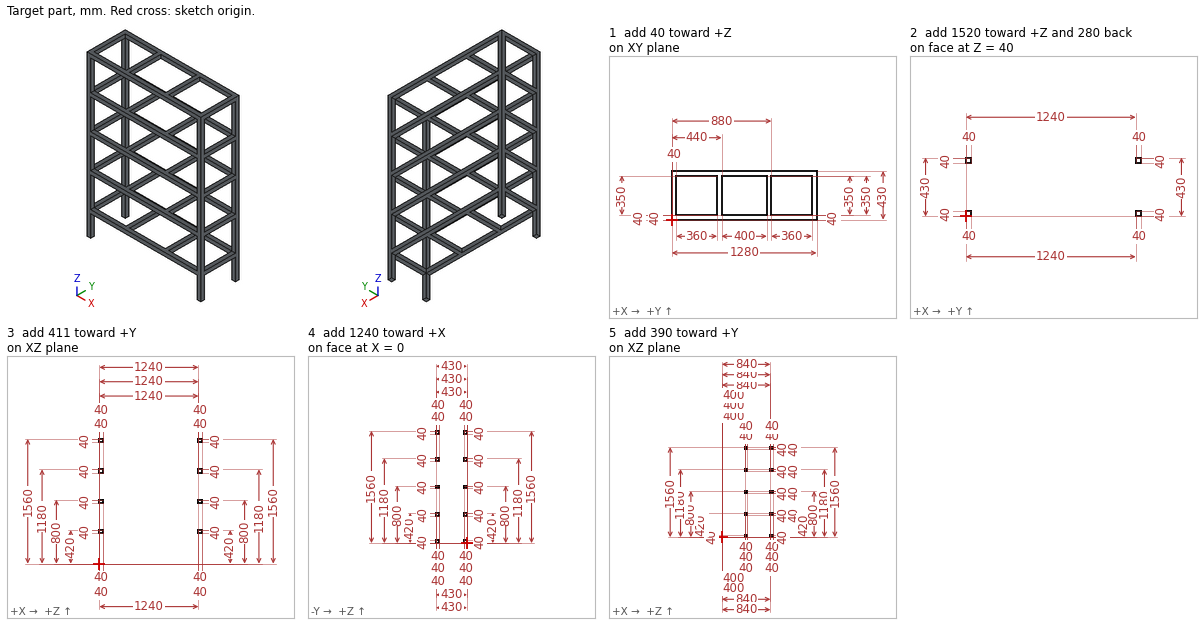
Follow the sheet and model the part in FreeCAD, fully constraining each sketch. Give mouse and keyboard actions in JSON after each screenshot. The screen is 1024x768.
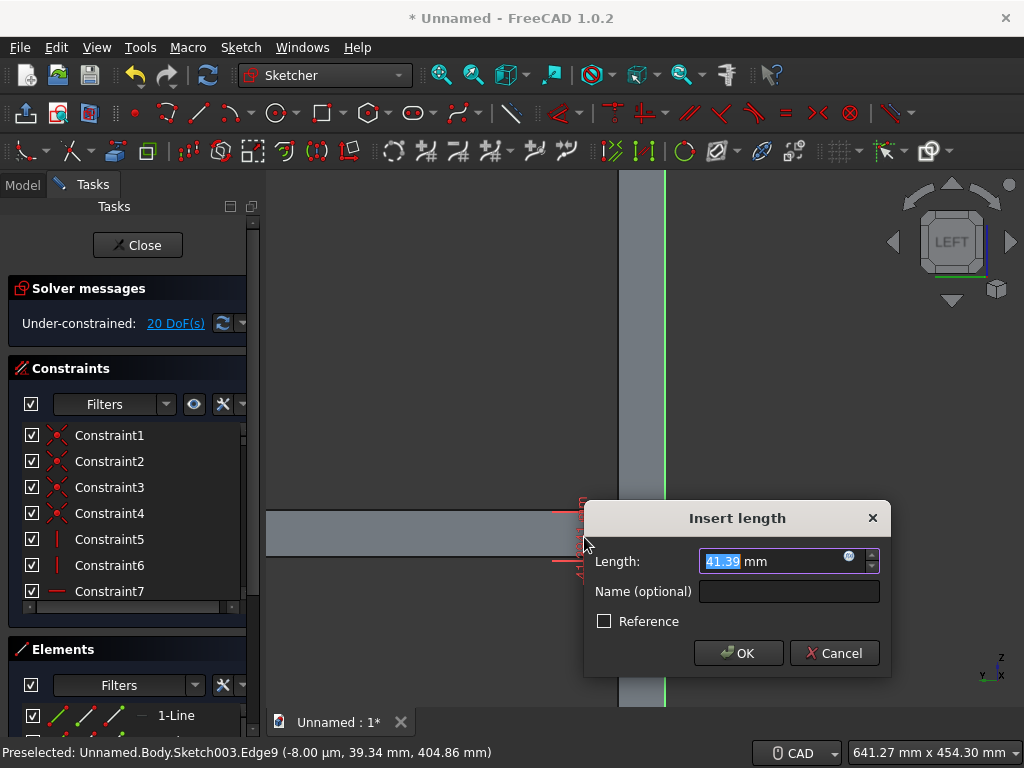
{"action": "type", "text": "40"}
{"action": "key", "text": "Return"}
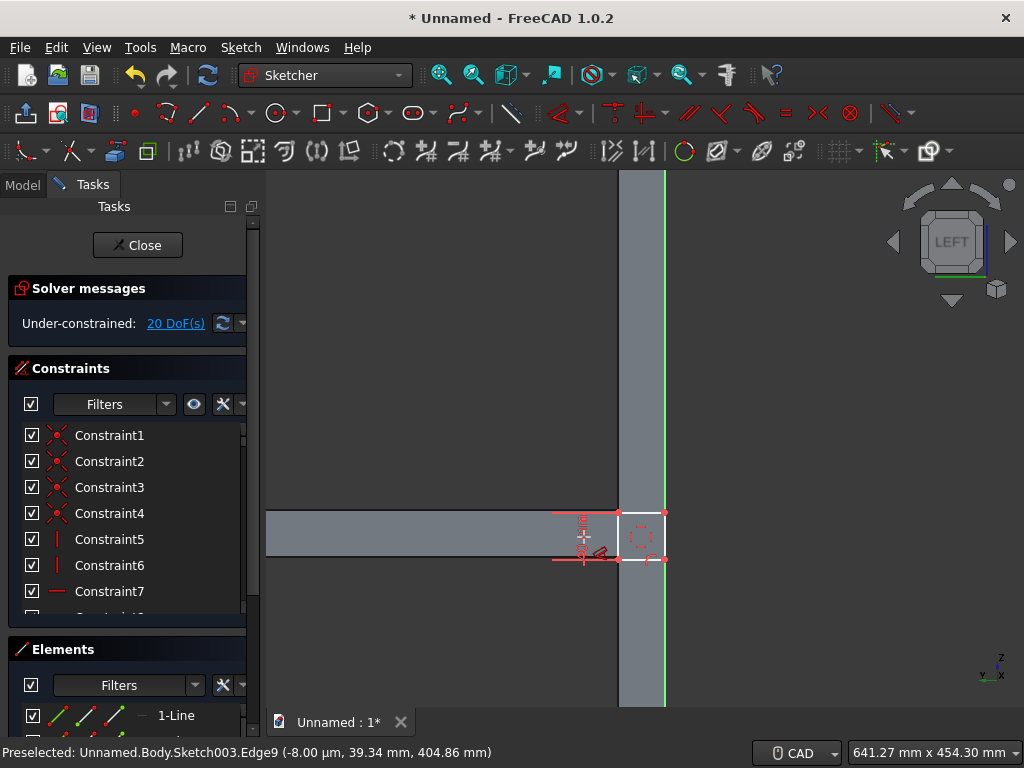
{"action": "left_click", "coordinate": [632, 560]}
{"action": "left_click", "coordinate": [642, 594]}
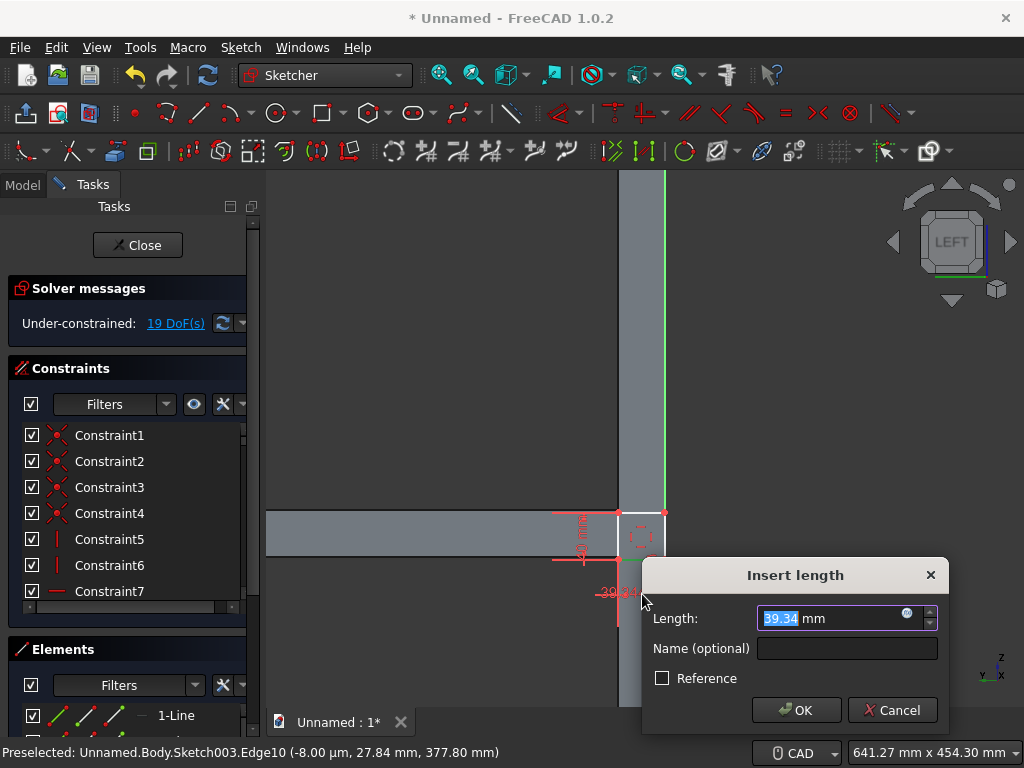
{"action": "type", "text": "40"}
{"action": "key", "text": "Return"}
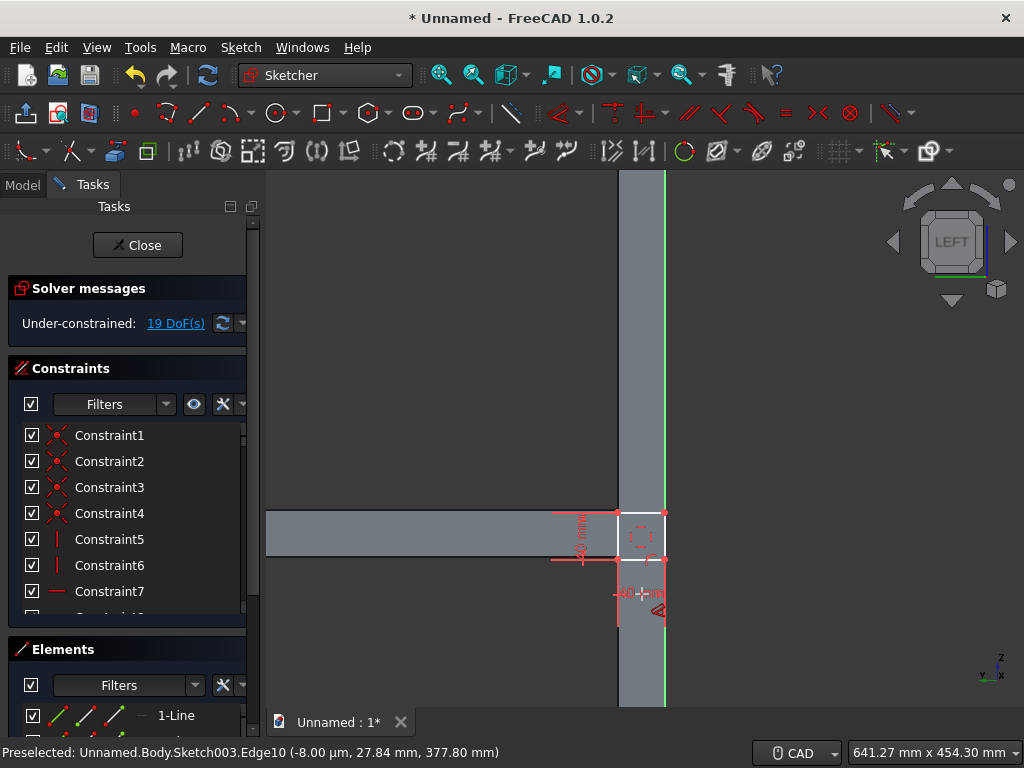
{"action": "scroll", "coordinate": [618, 528], "scroll_direction": "down", "scroll_amount": 8}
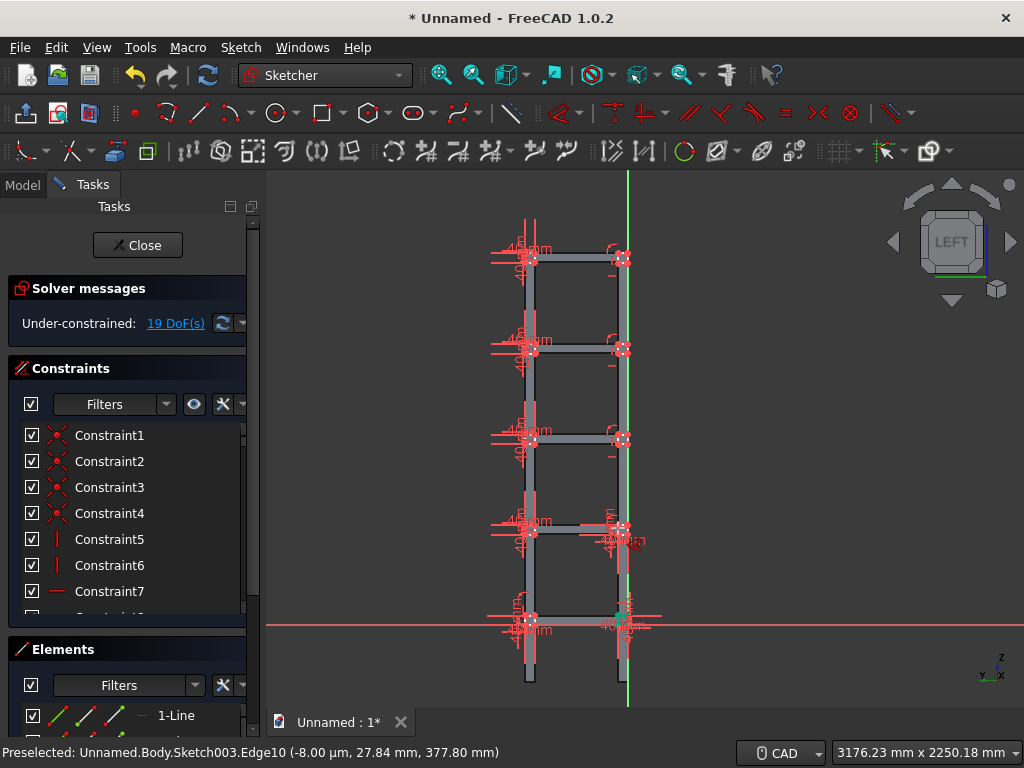
{"action": "scroll", "coordinate": [618, 438], "scroll_direction": "up", "scroll_amount": 8}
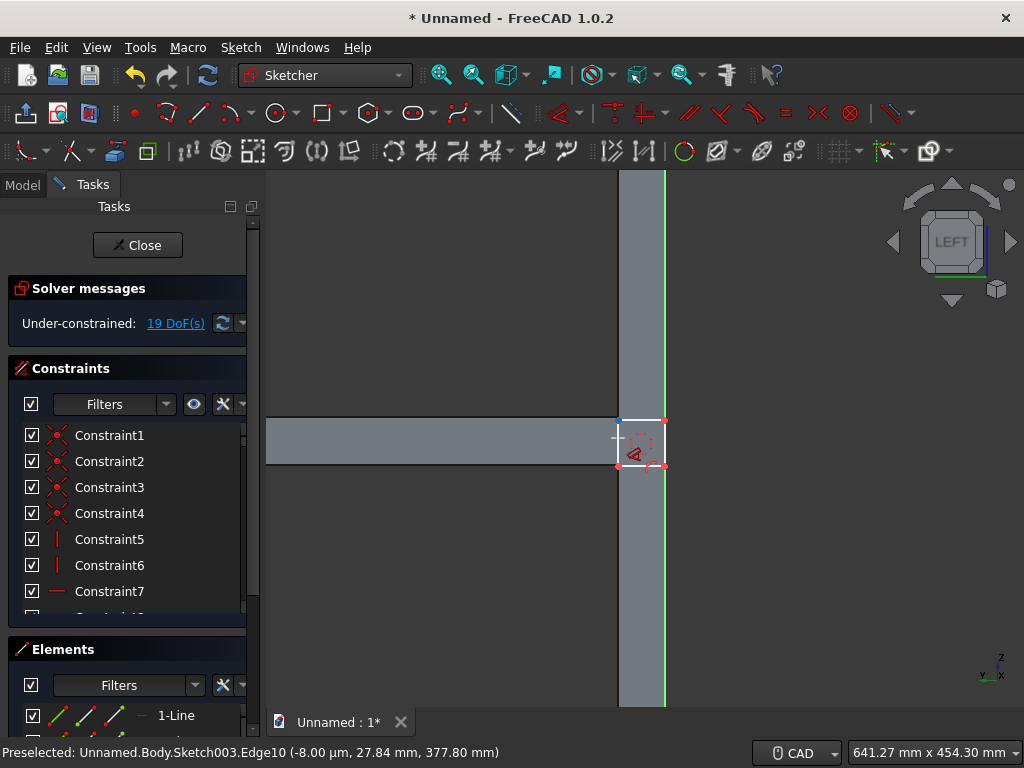
{"action": "left_click", "coordinate": [618, 434]}
{"action": "left_click", "coordinate": [584, 443]}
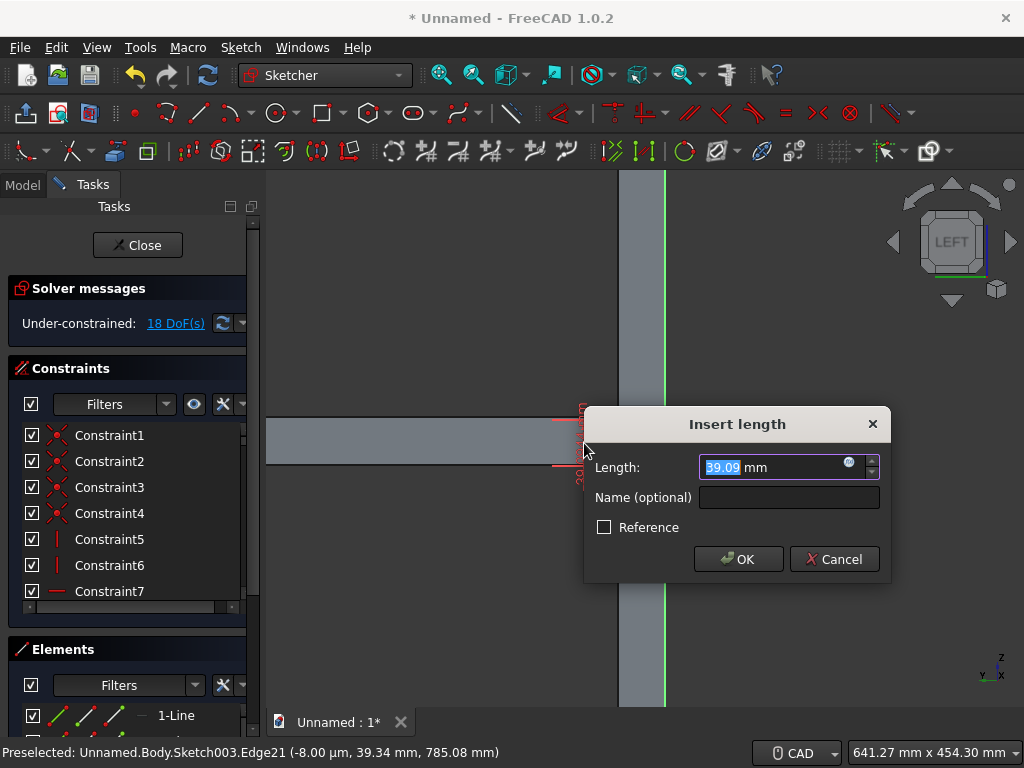
{"action": "type", "text": "40"}
{"action": "key", "text": "Return"}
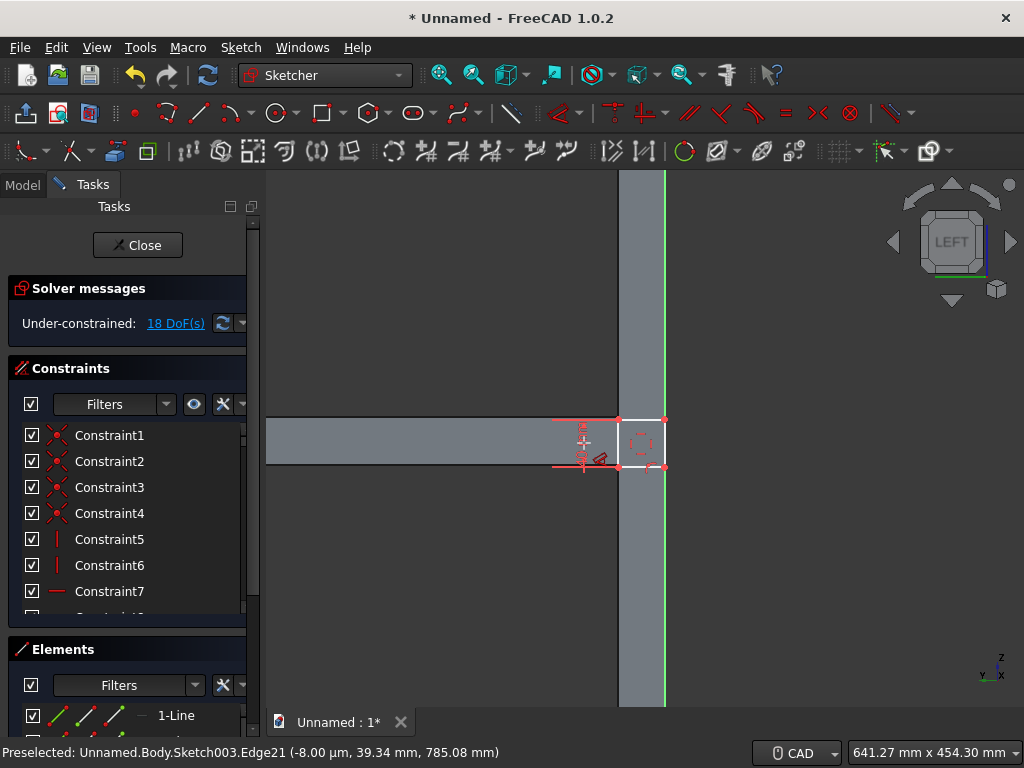
{"action": "left_click", "coordinate": [632, 467]}
{"action": "left_click", "coordinate": [642, 501]}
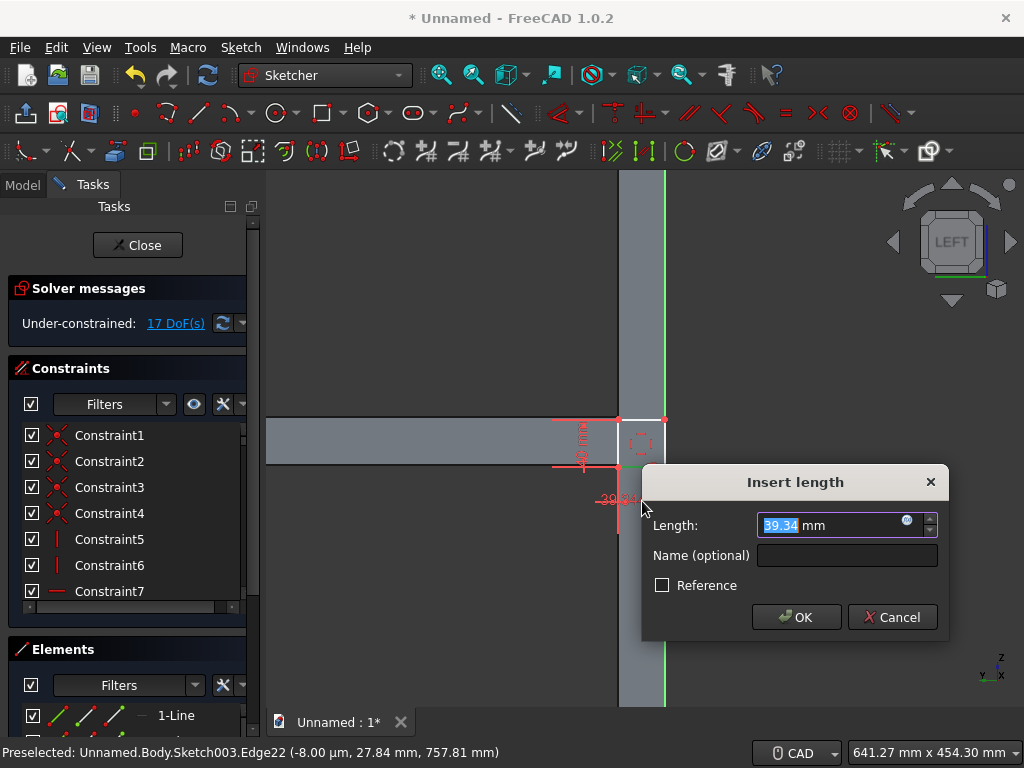
{"action": "type", "text": "40"}
{"action": "key", "text": "Return"}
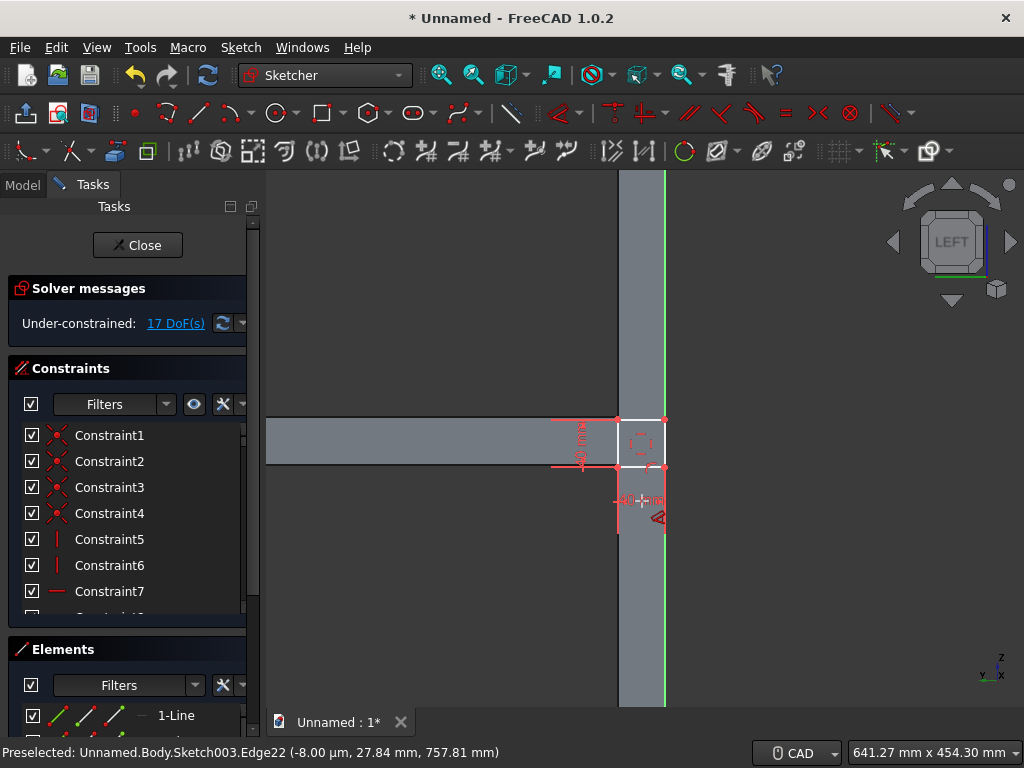
{"action": "scroll", "coordinate": [618, 438], "scroll_direction": "down", "scroll_amount": 8}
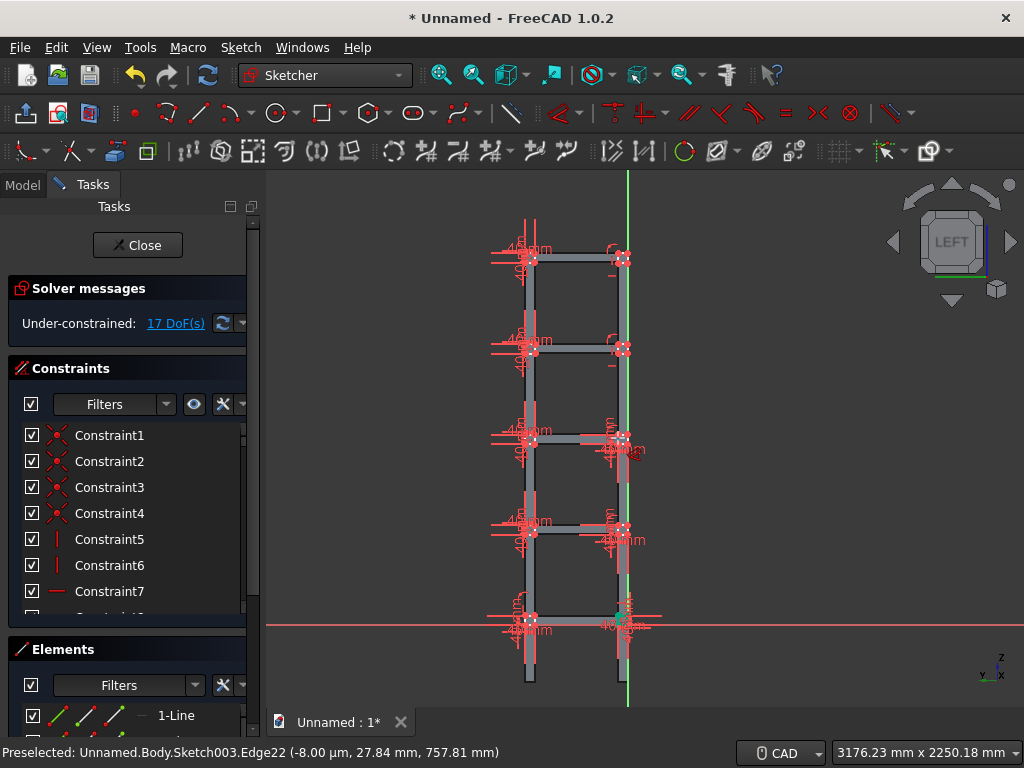
{"action": "scroll", "coordinate": [618, 347], "scroll_direction": "up", "scroll_amount": 8}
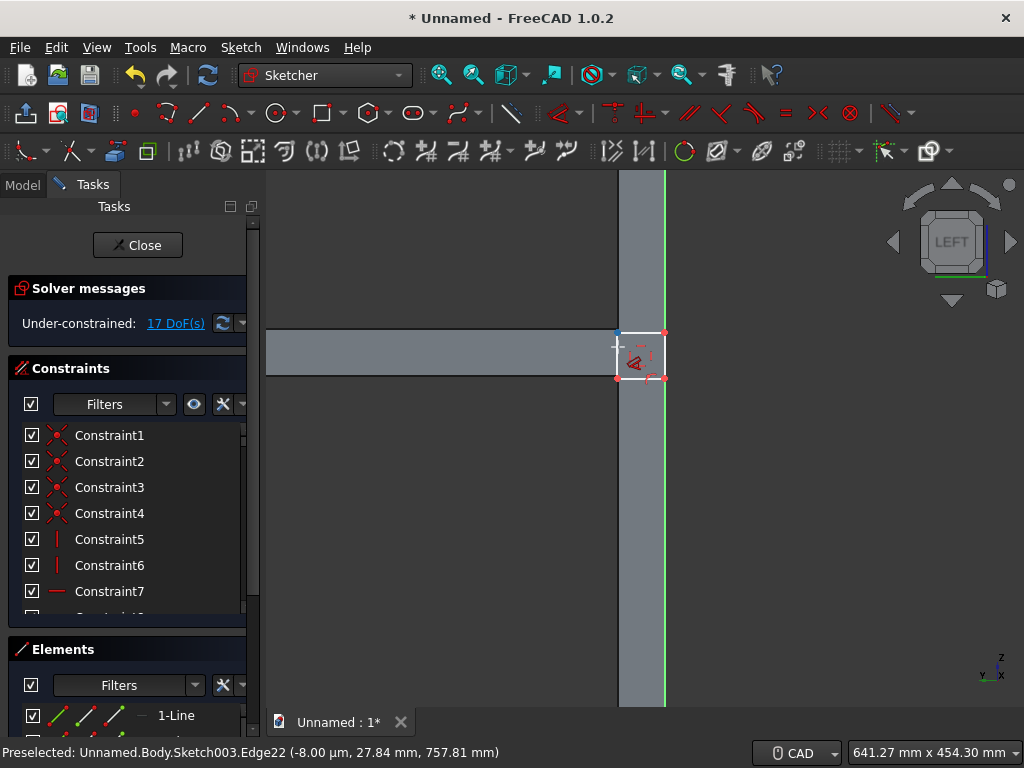
{"action": "left_click", "coordinate": [617, 346]}
{"action": "left_click", "coordinate": [651, 356]}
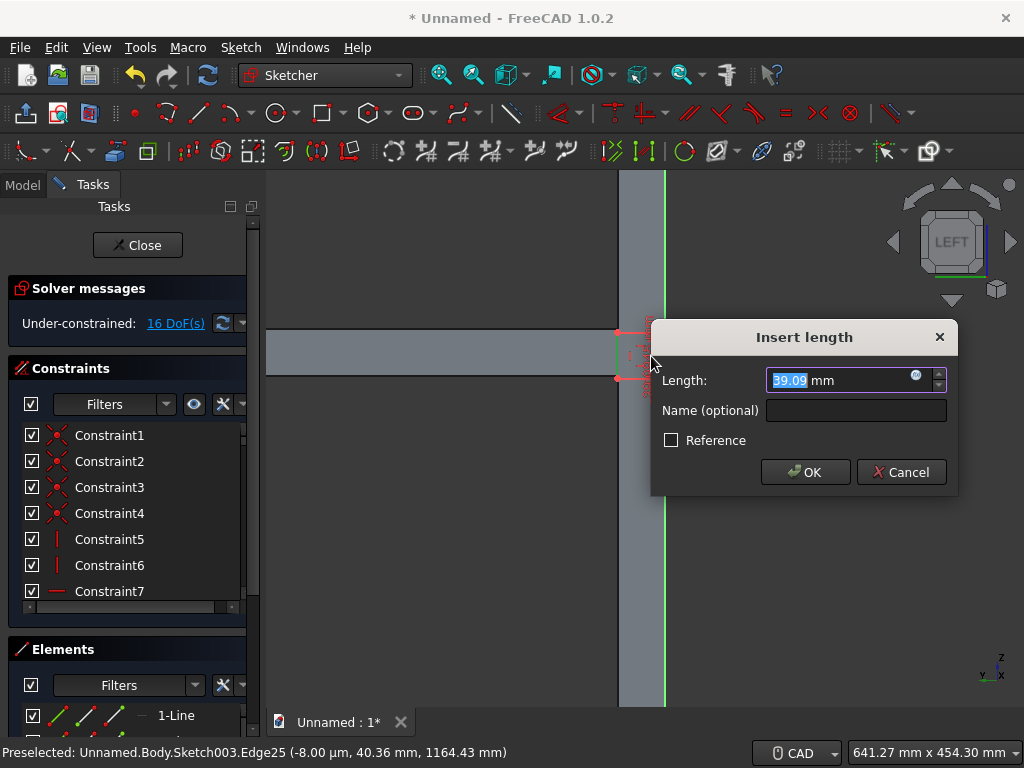
{"action": "type", "text": "40"}
{"action": "key", "text": "Return"}